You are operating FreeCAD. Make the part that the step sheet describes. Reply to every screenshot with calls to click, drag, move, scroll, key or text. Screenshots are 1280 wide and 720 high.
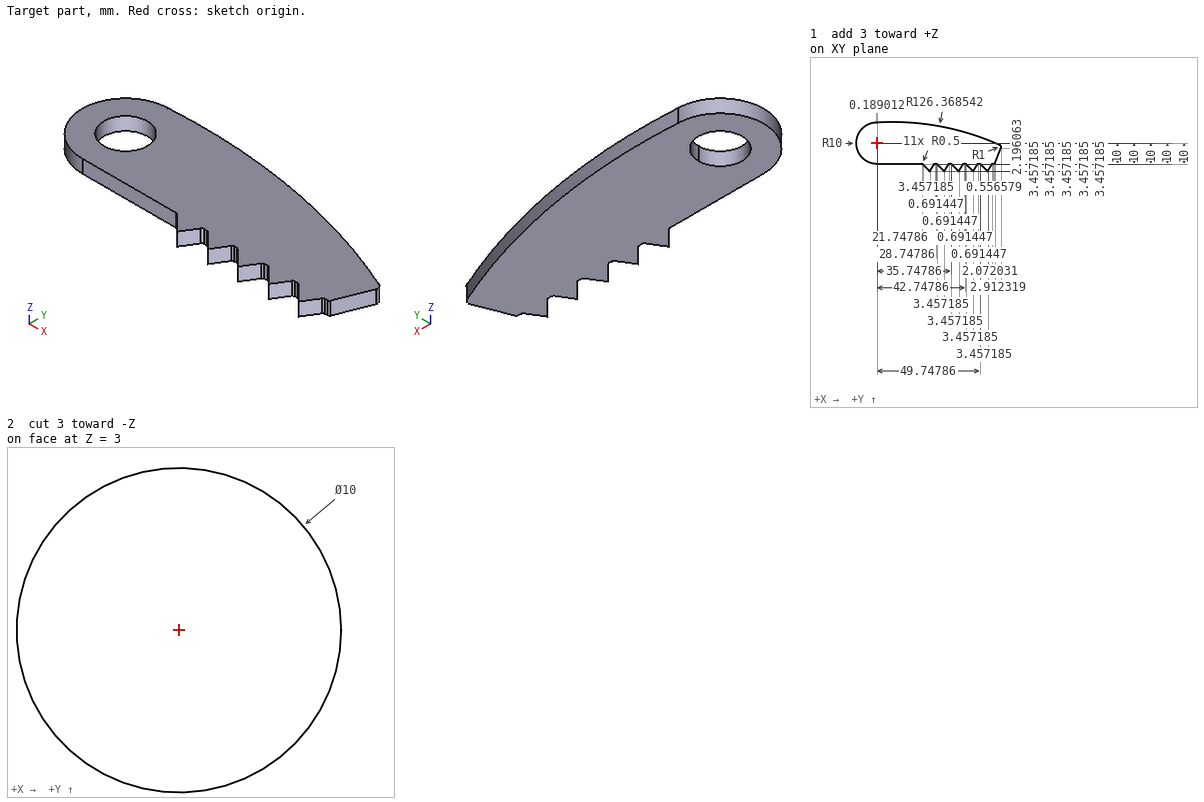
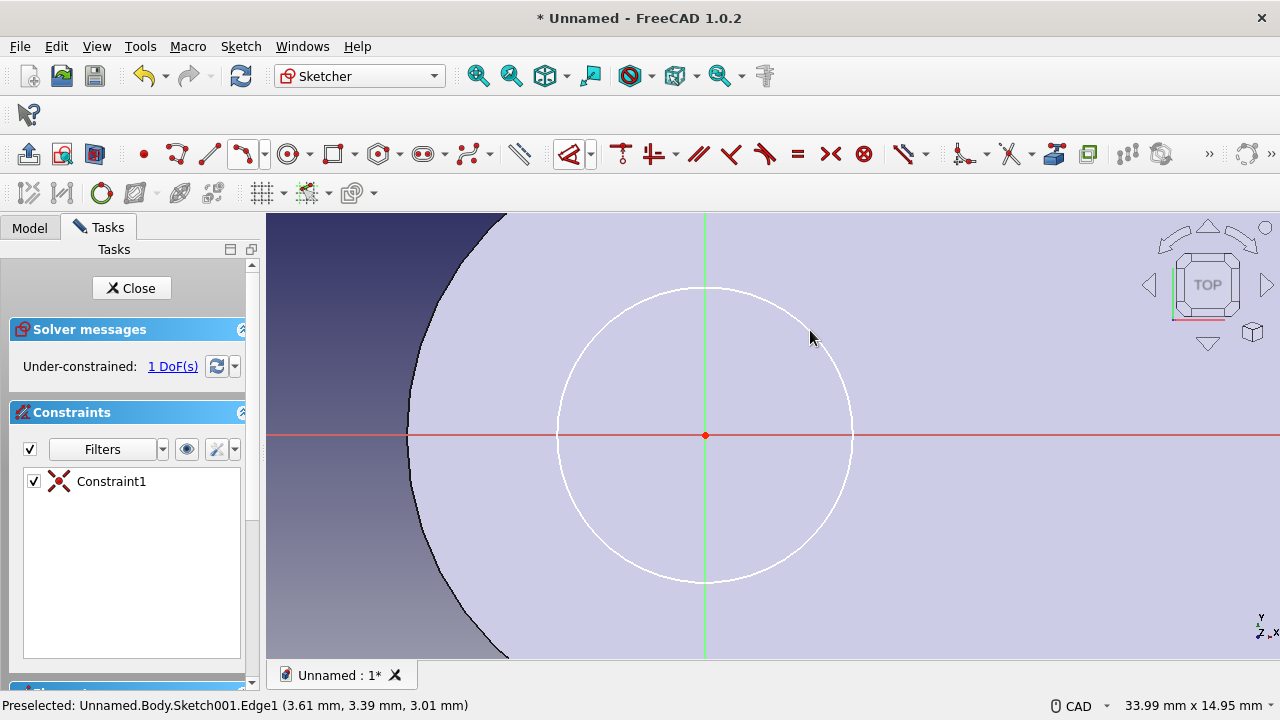
click(809, 330)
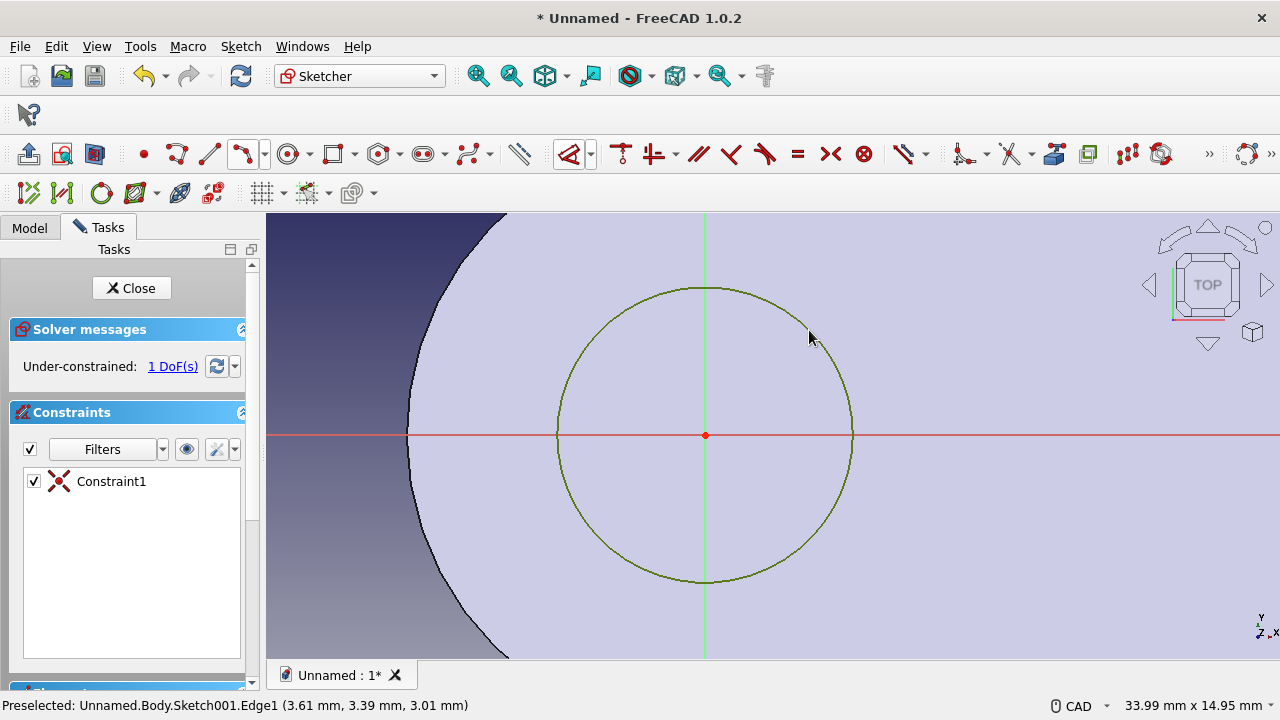
key(k)
key(o)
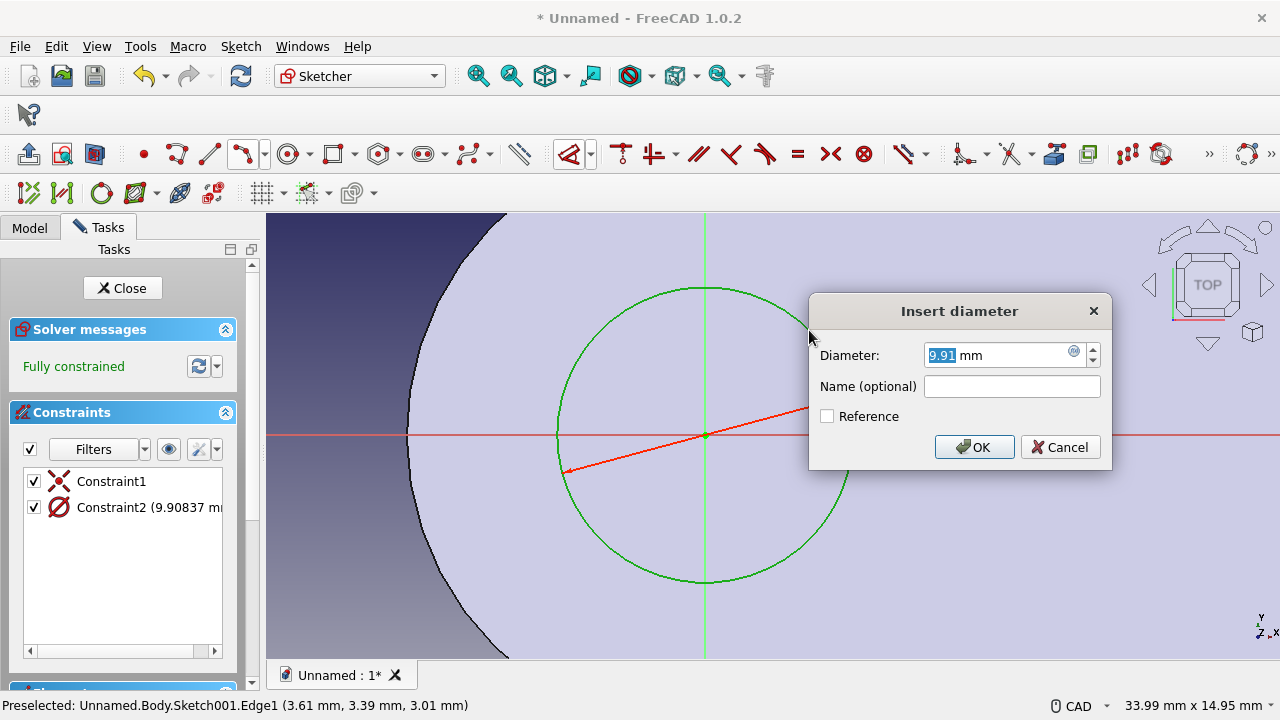
text(10)
key(Return)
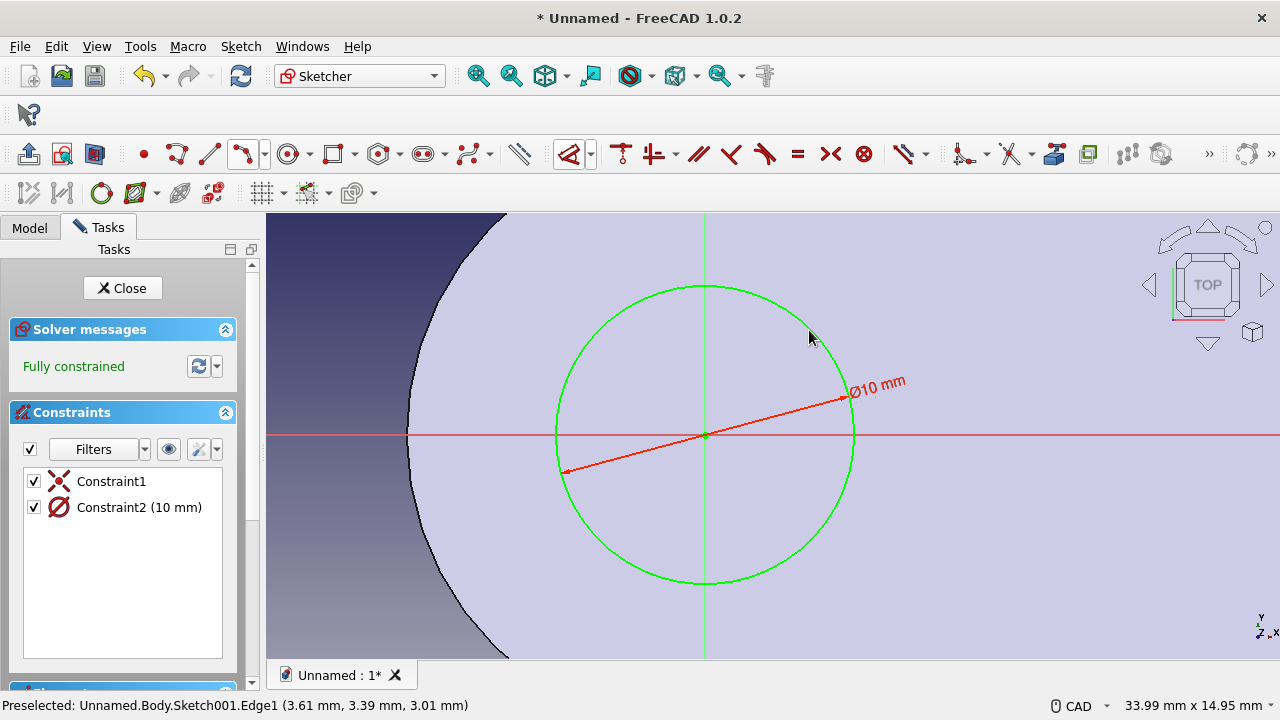
click(123, 288)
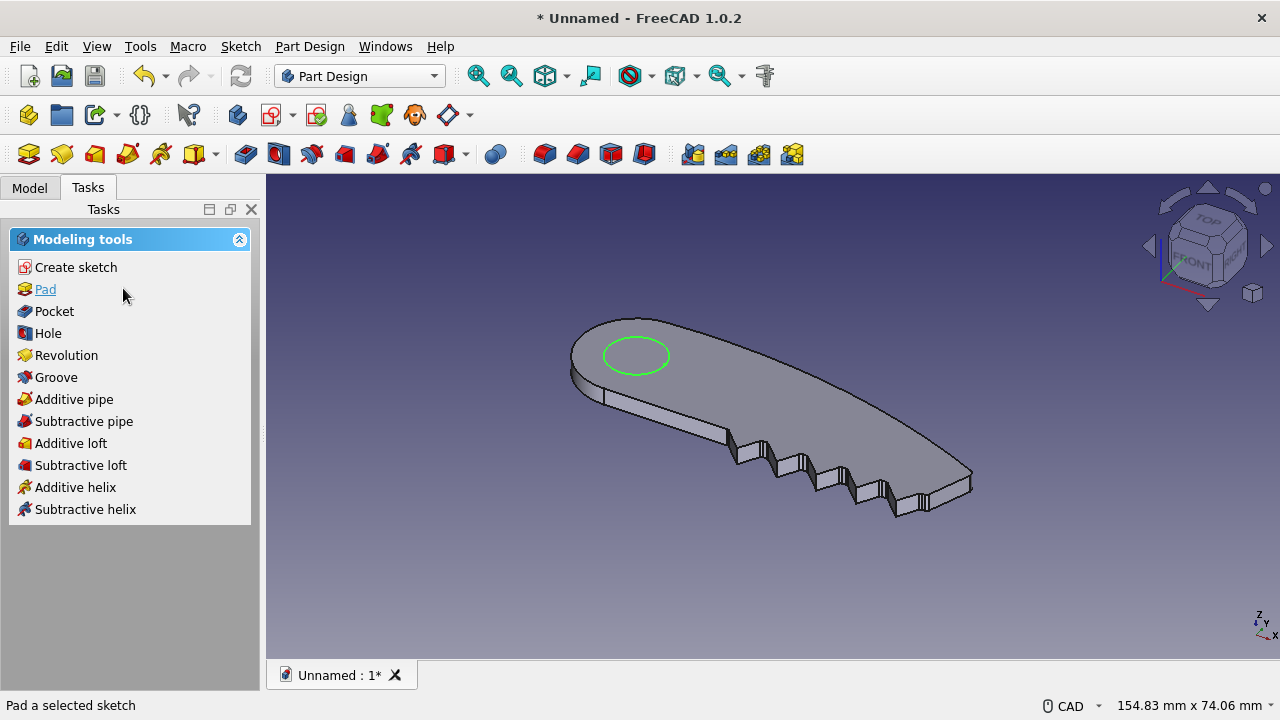
click(246, 154)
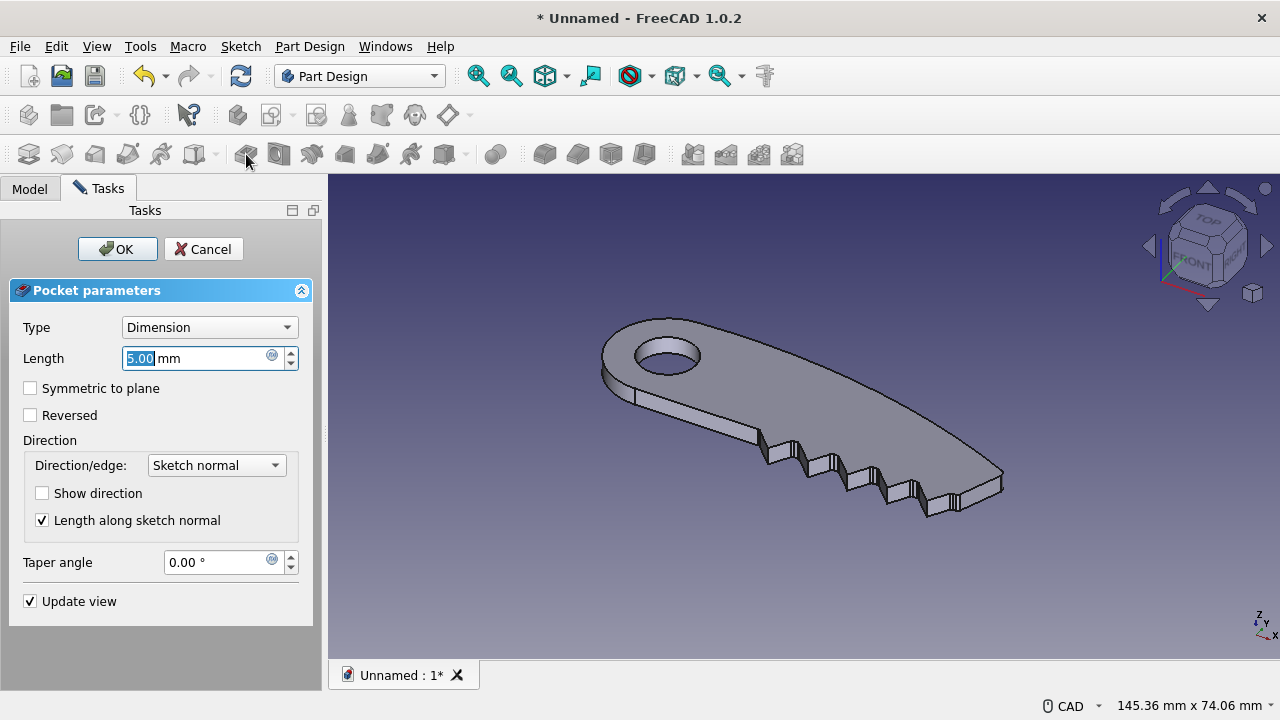
text(3)
key(Tab)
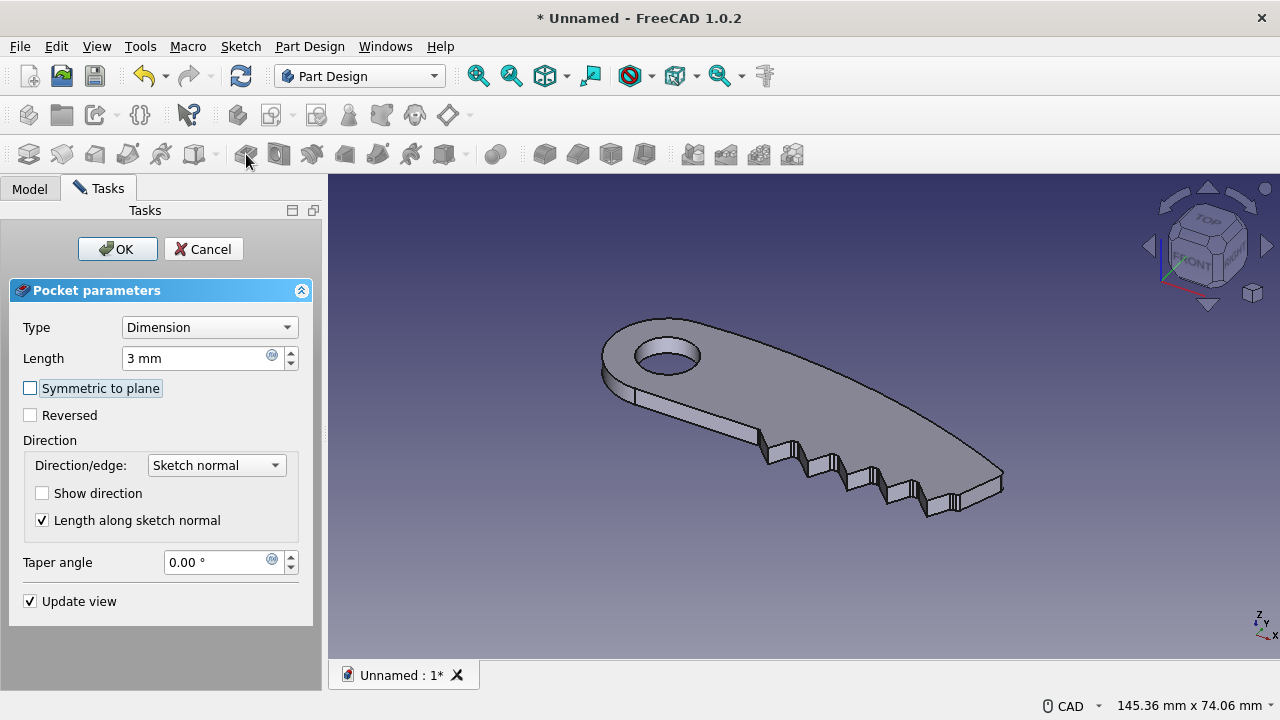
click(118, 249)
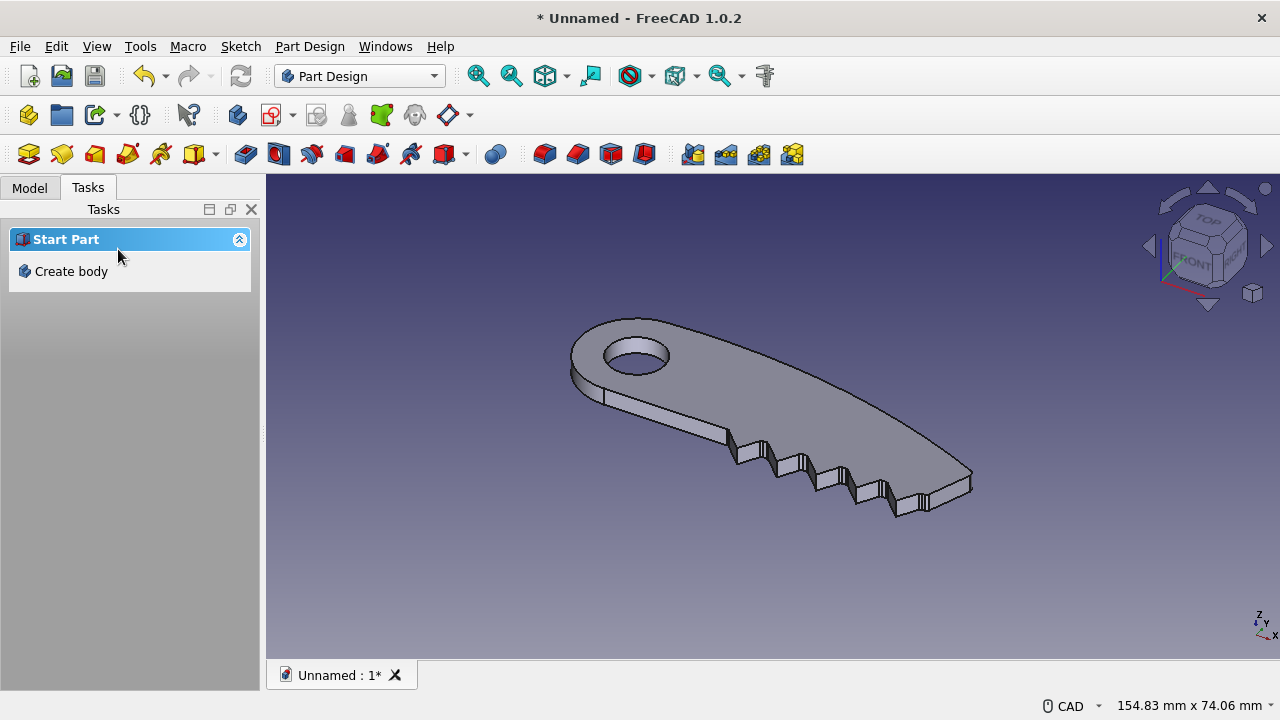
key(0)